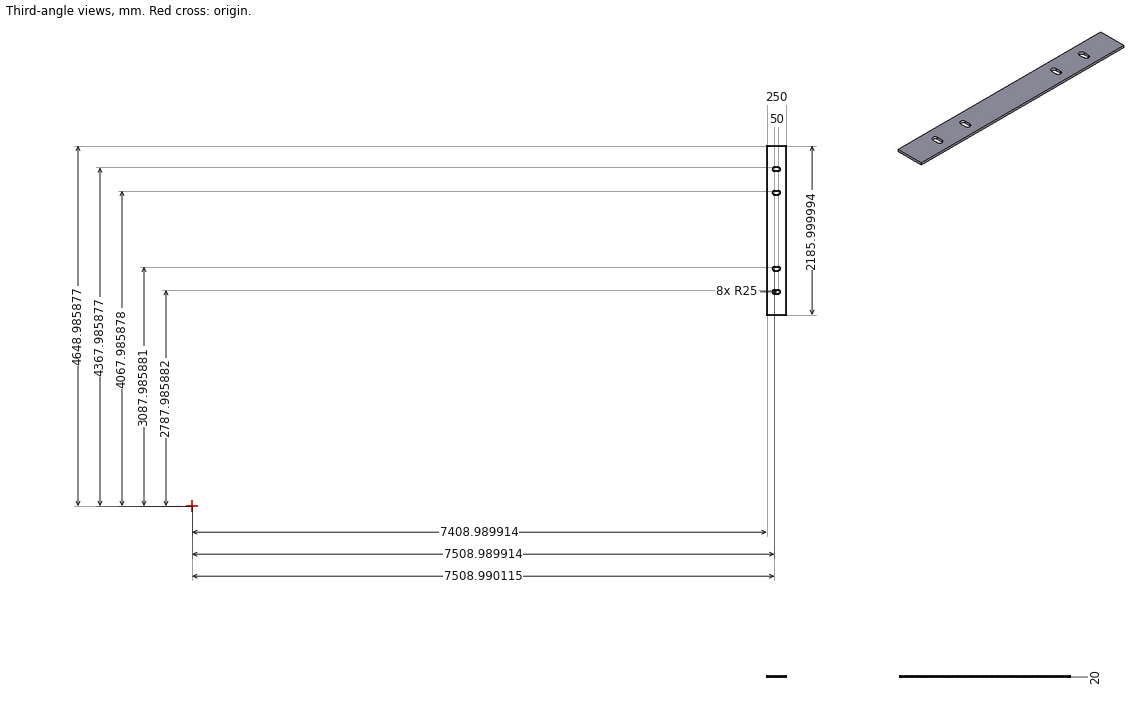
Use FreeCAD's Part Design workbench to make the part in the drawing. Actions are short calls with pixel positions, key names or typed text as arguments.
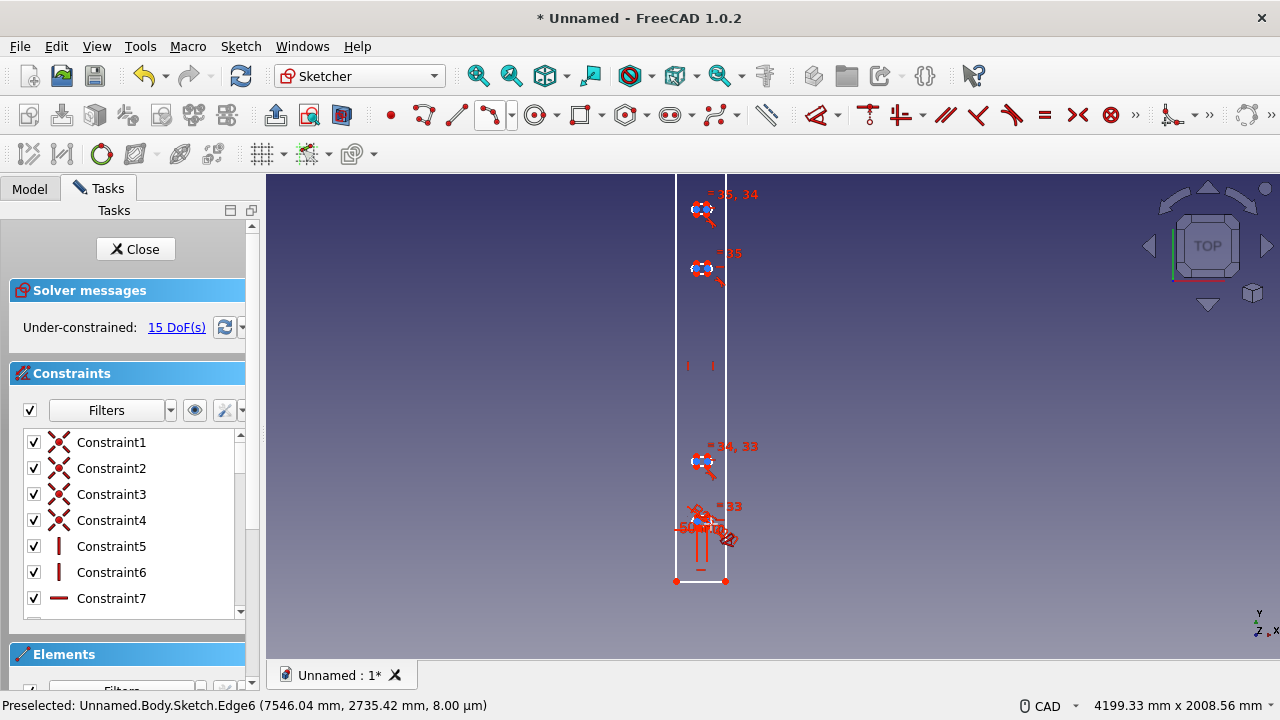
scroll(706, 486, up, 10)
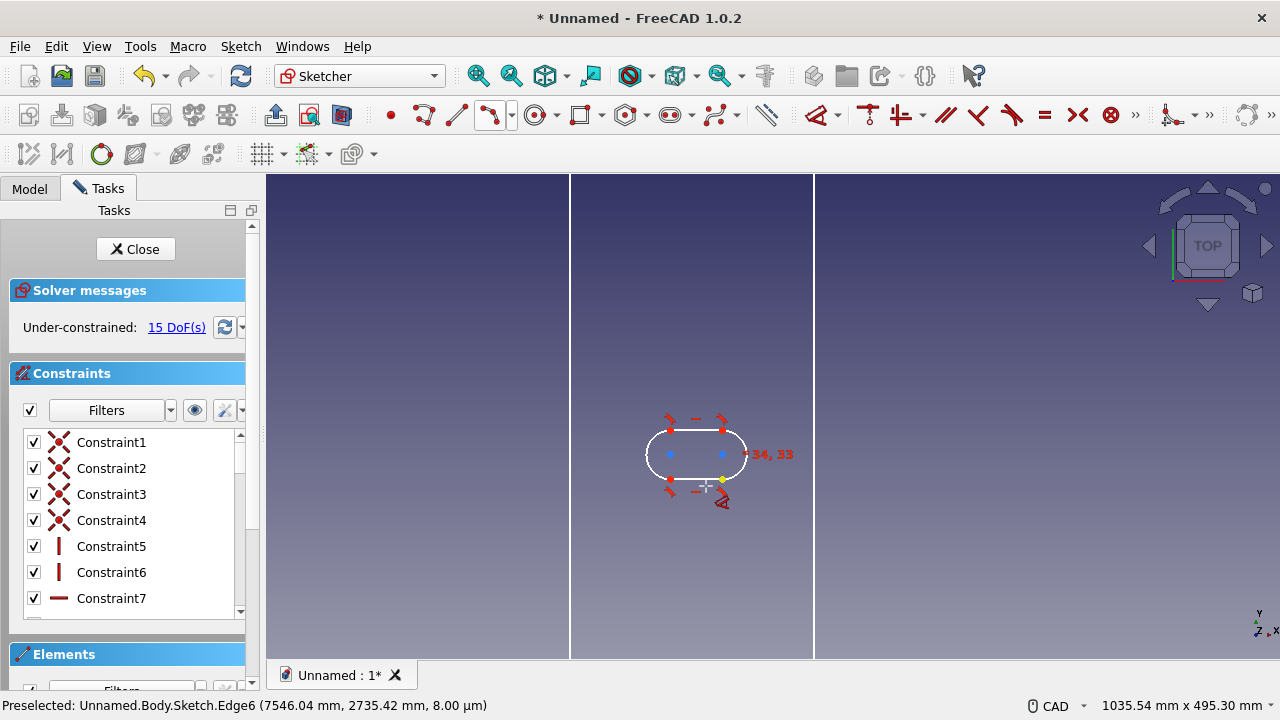
click(707, 479)
click(697, 513)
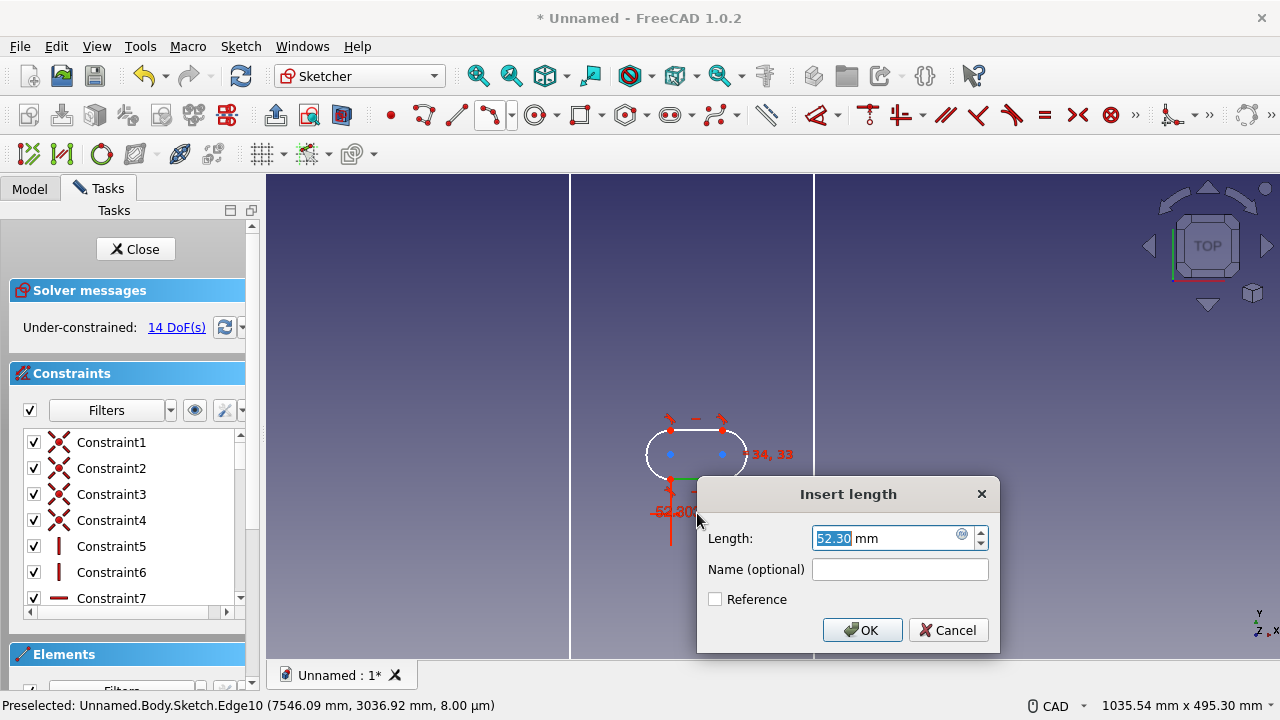
text(50)
key(Return)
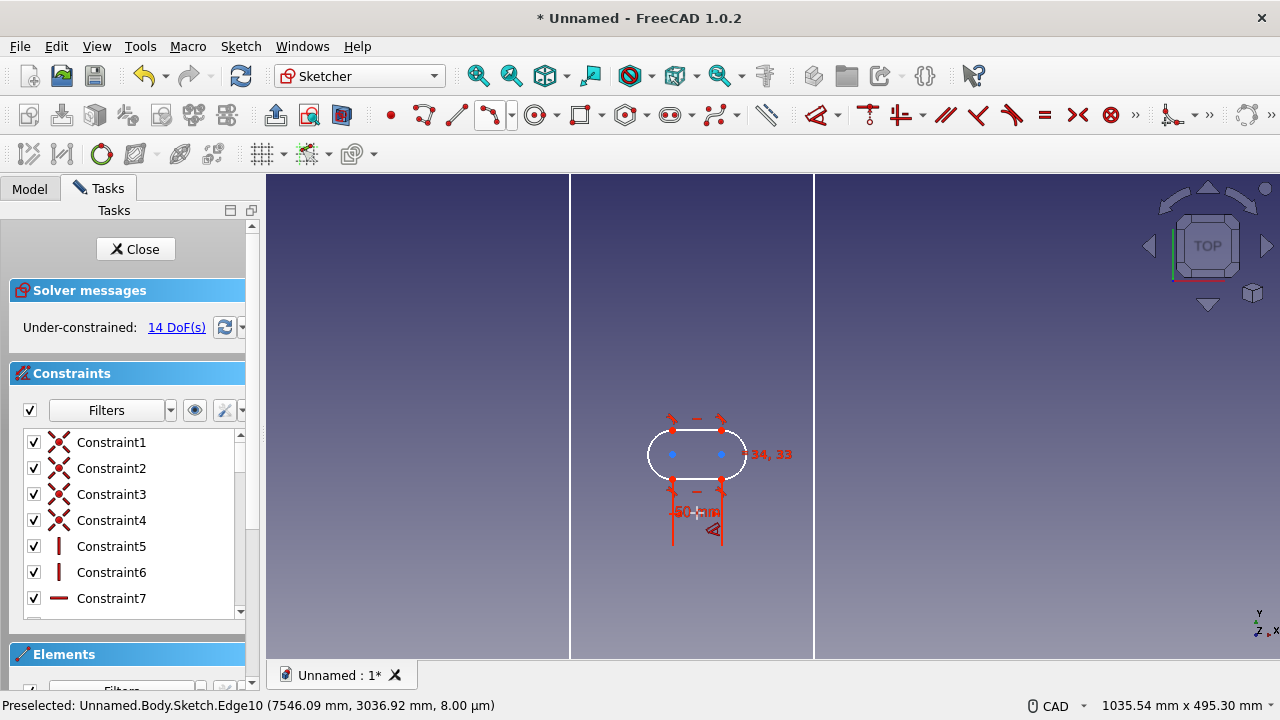
scroll(706, 486, down, 10)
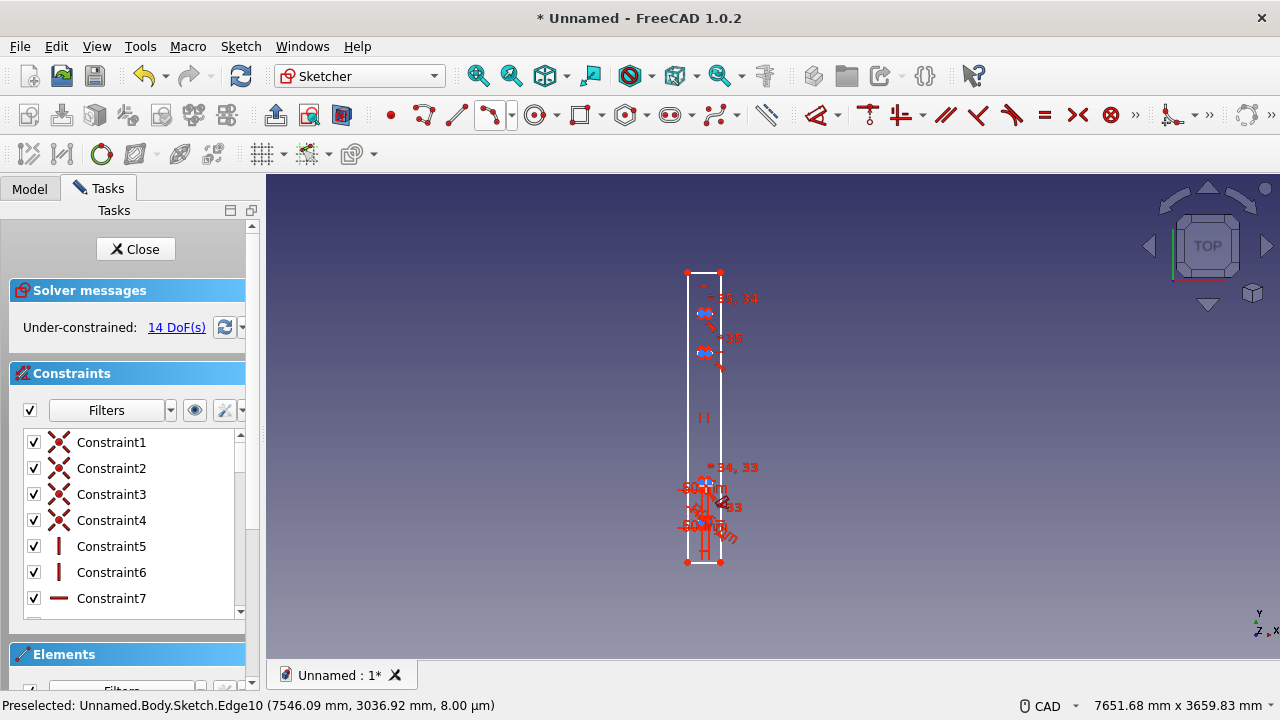
scroll(704, 310, up, 10)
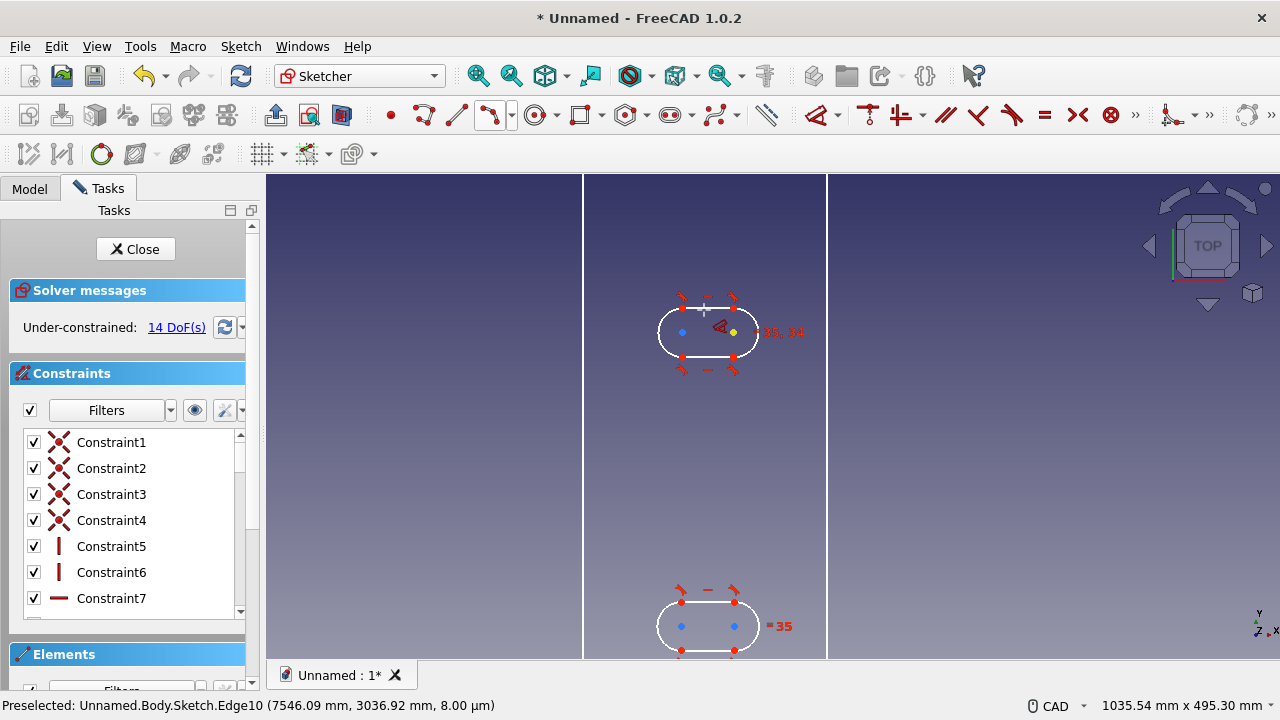
click(698, 308)
click(708, 274)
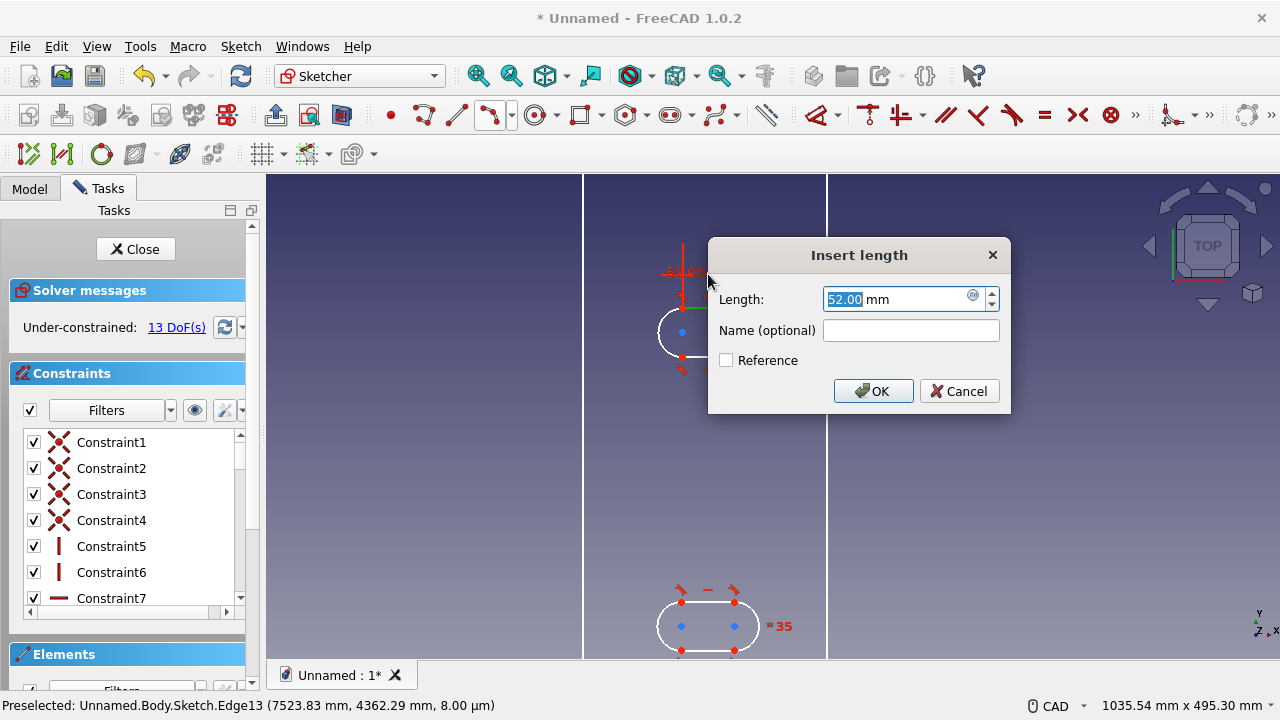
text(50)
key(Return)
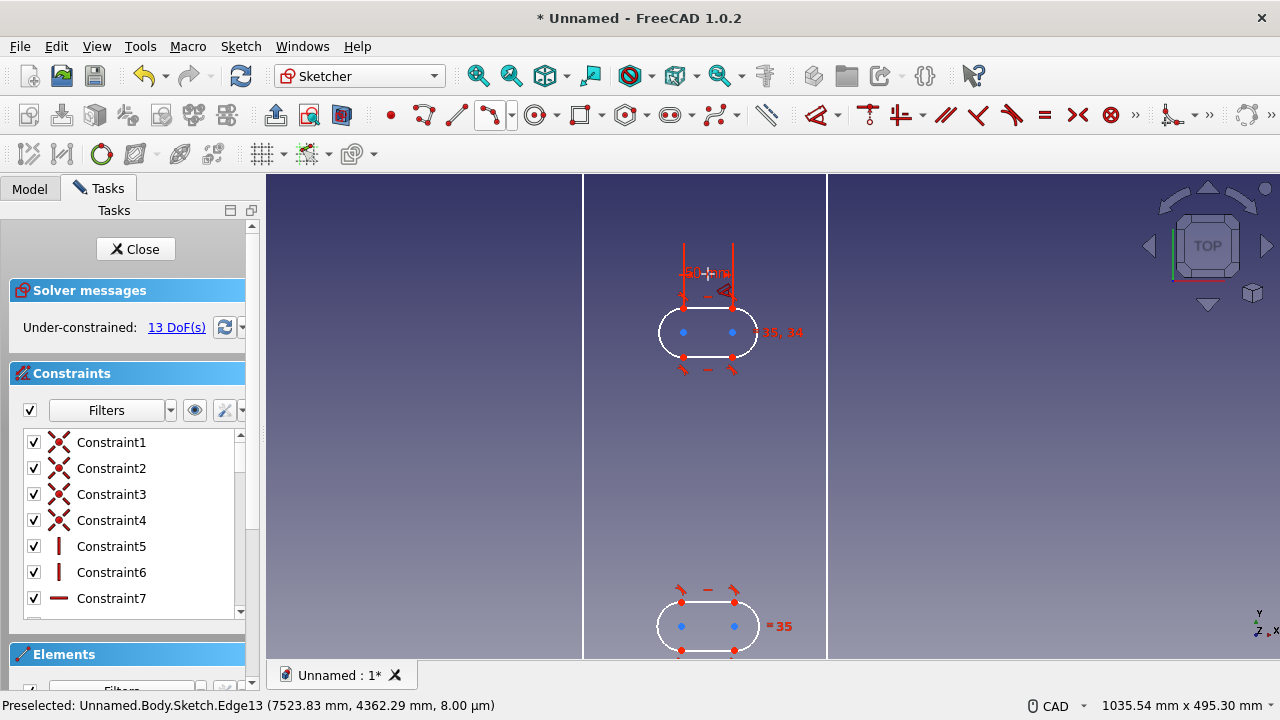
click(698, 602)
click(708, 568)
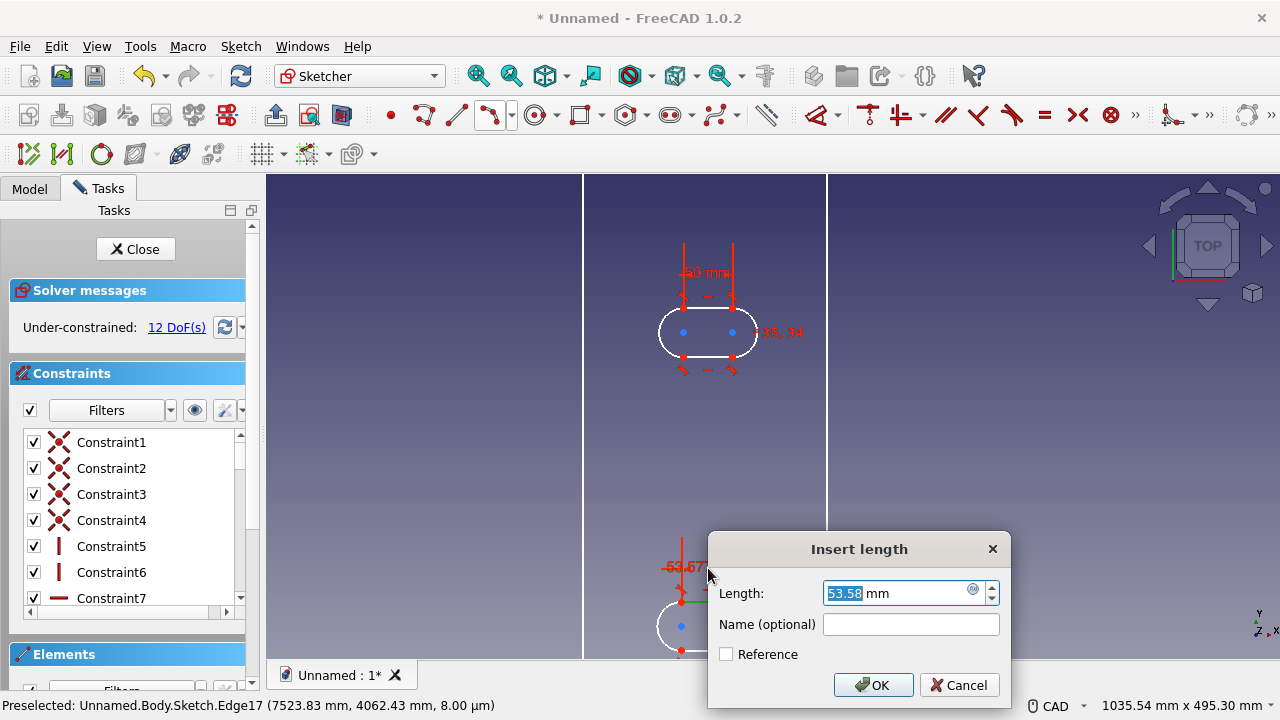
text(50)
key(Return)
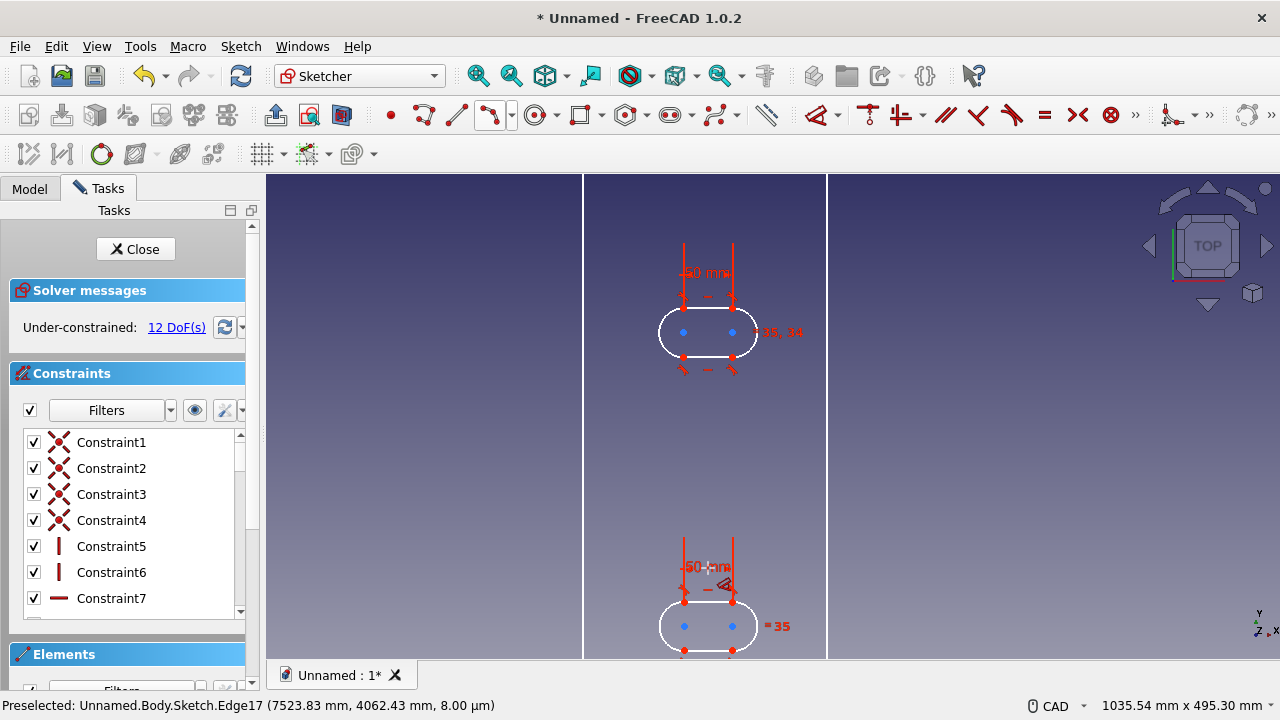
scroll(704, 310, down, 10)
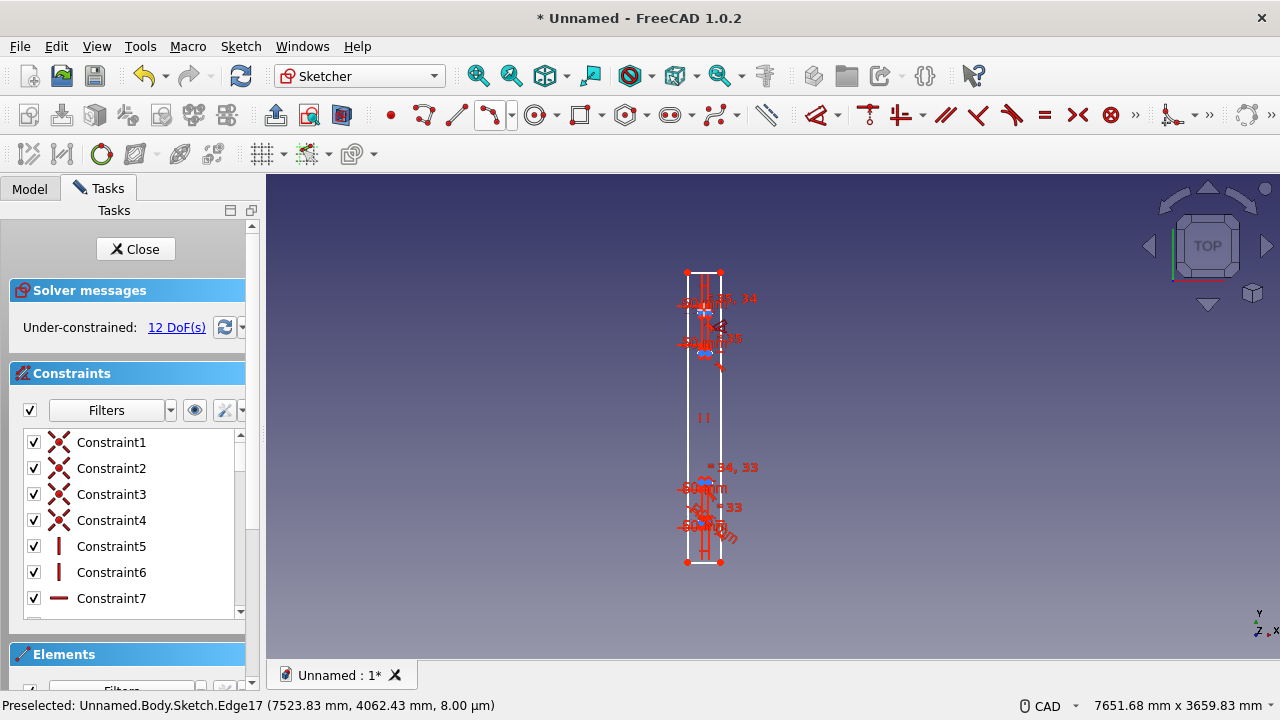
scroll(698, 563, up, 2)